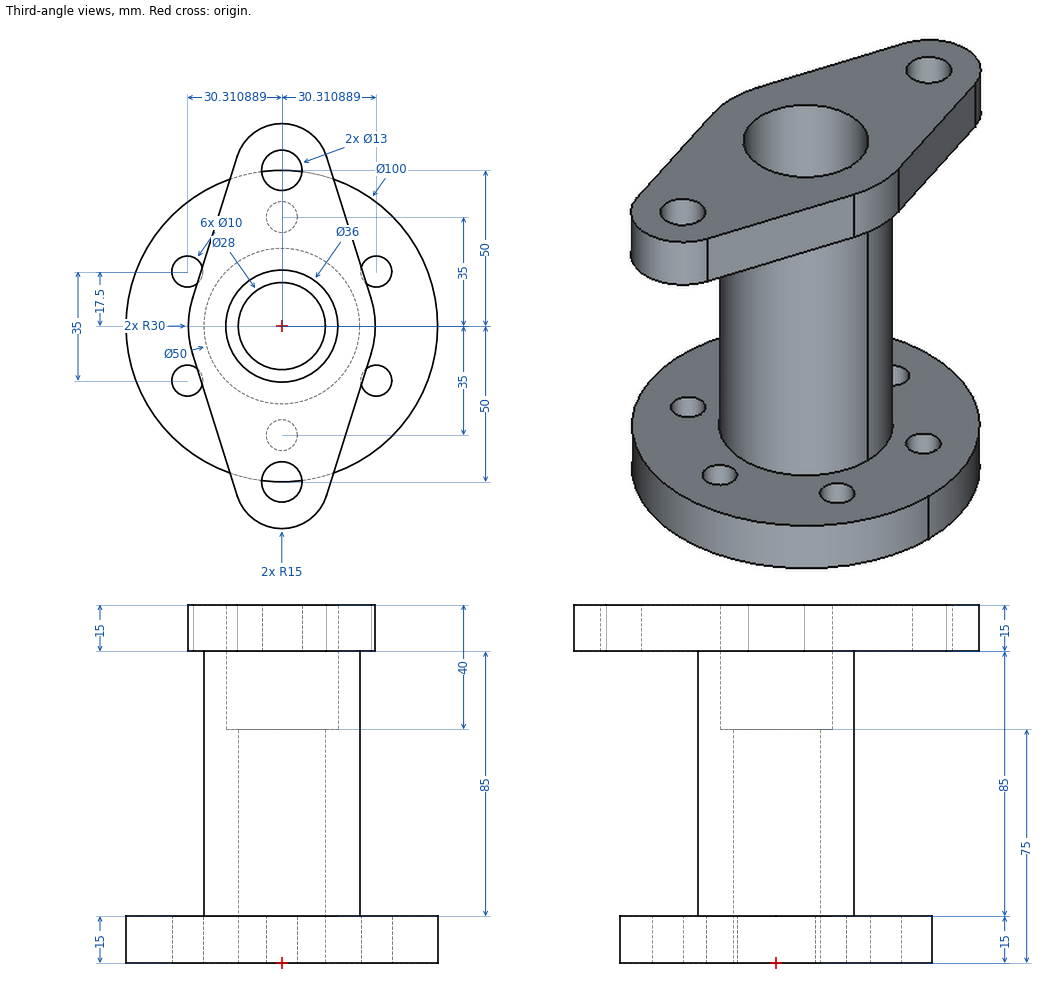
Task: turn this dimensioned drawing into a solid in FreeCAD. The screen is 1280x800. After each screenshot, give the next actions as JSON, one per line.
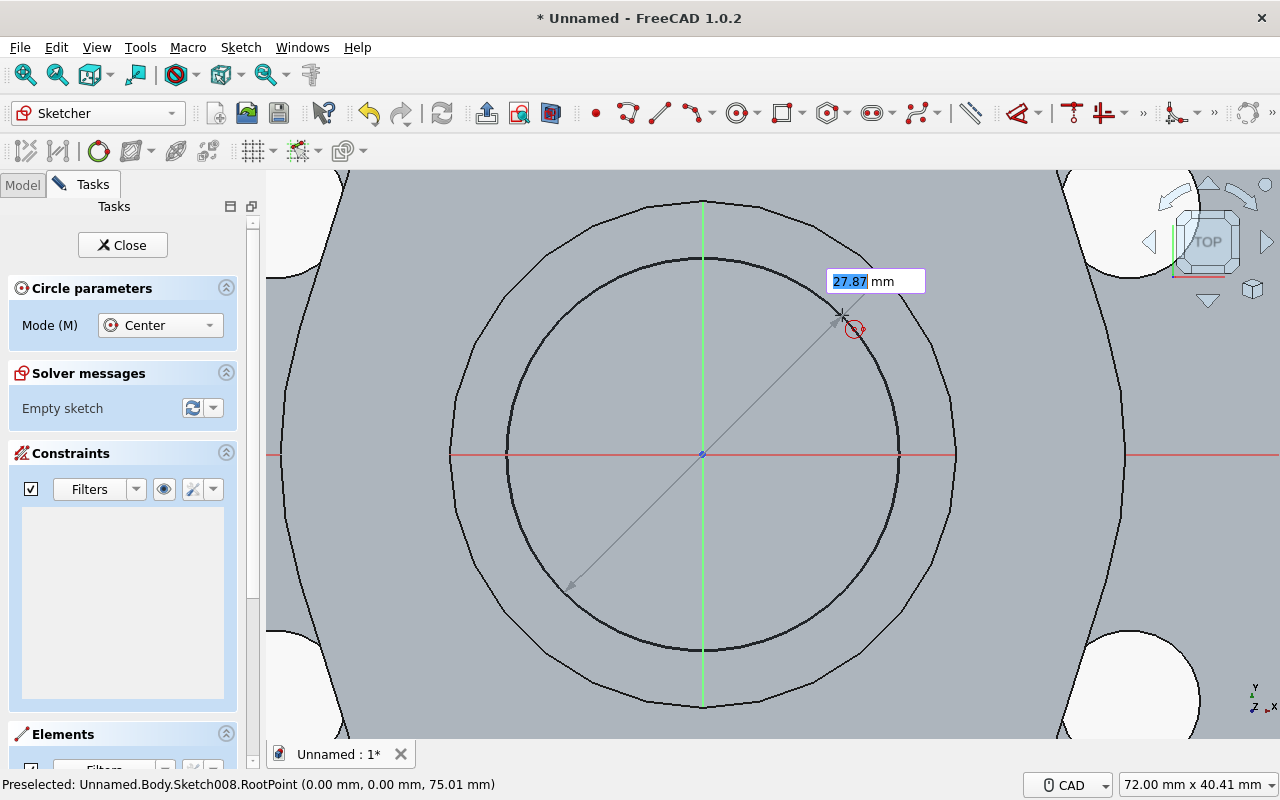
{"action": "type", "text": "28"}
{"action": "key", "text": "Return"}
{"action": "key", "text": "Escape"}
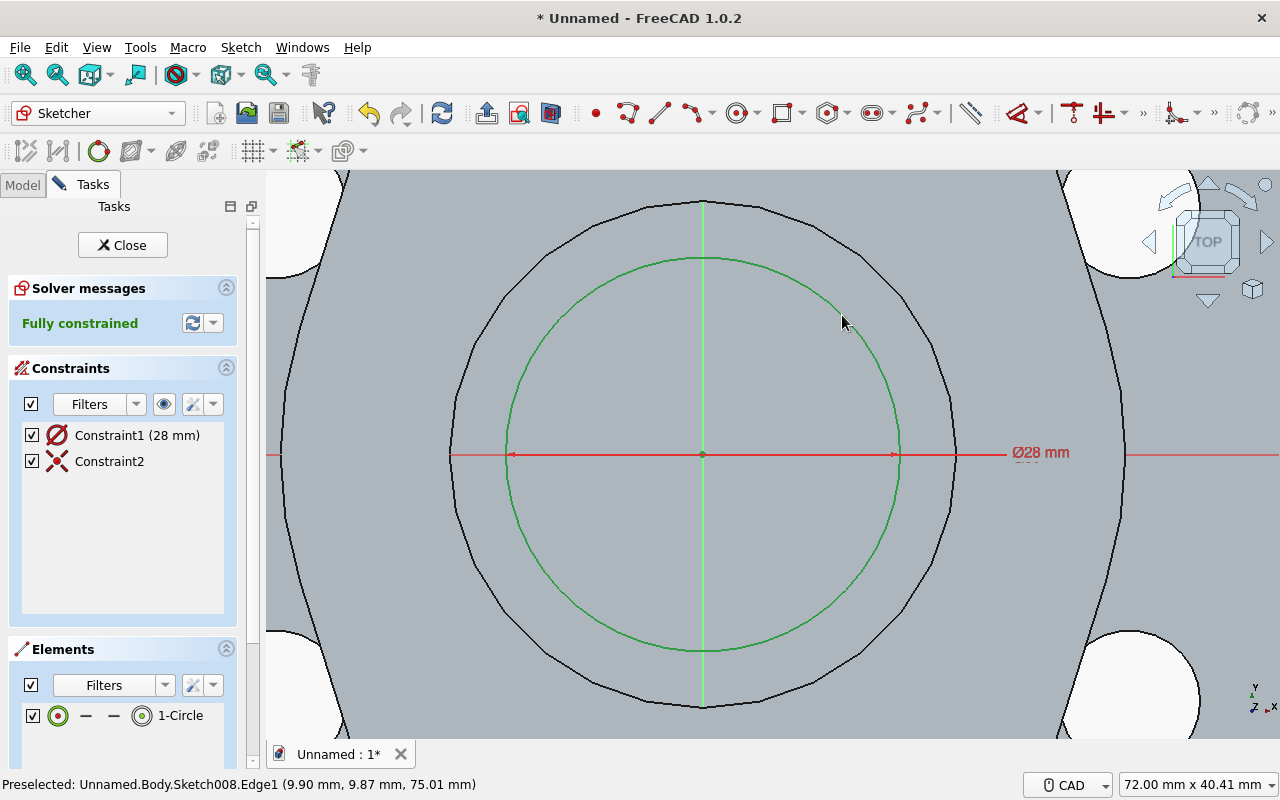
{"action": "left_click", "coordinate": [123, 245]}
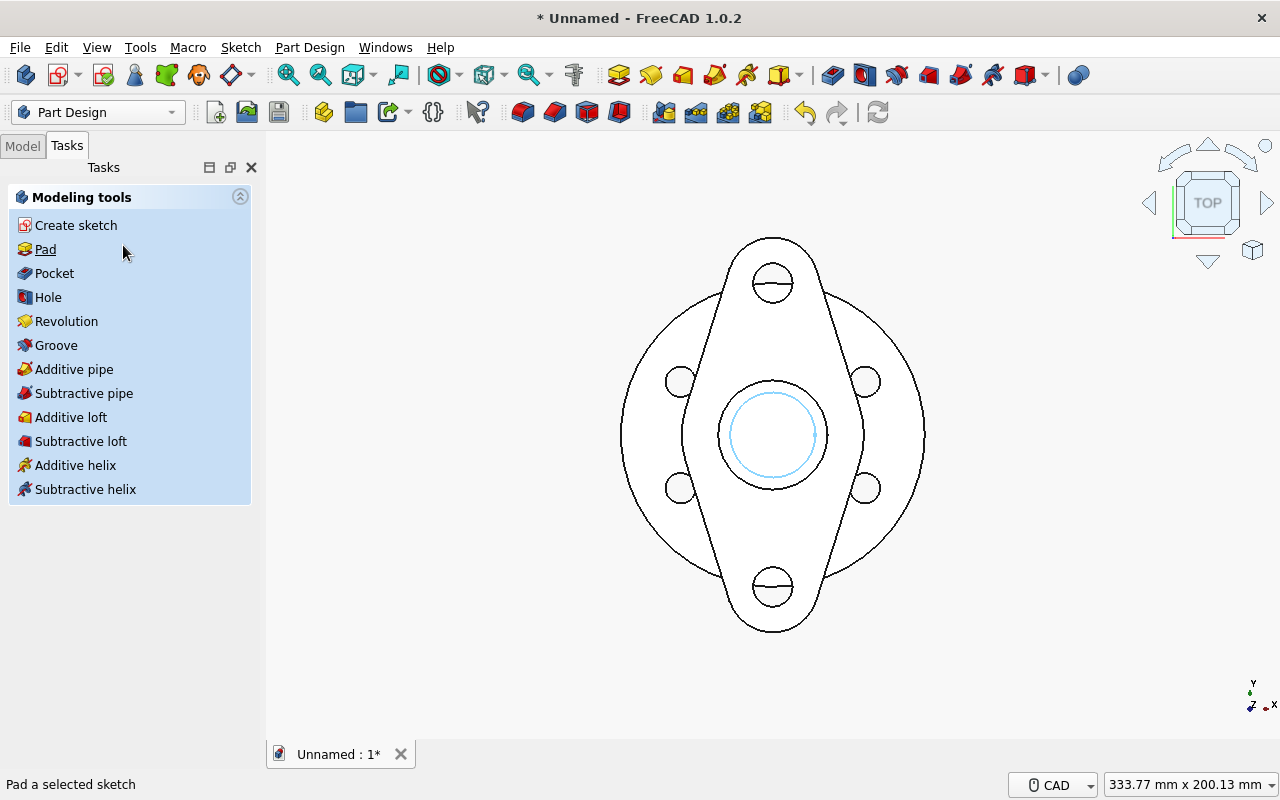
{"action": "left_click", "coordinate": [834, 76]}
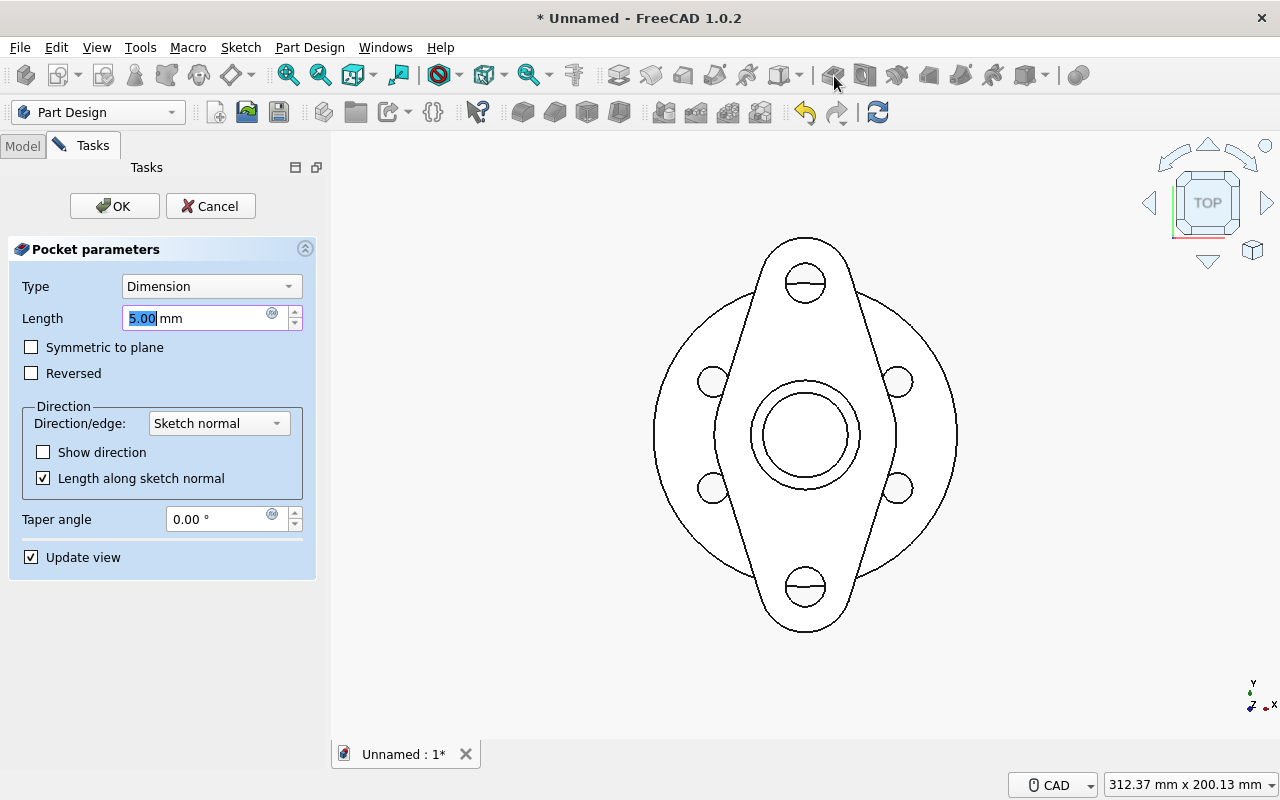
{"action": "type", "text": "75"}
{"action": "key", "text": "Tab"}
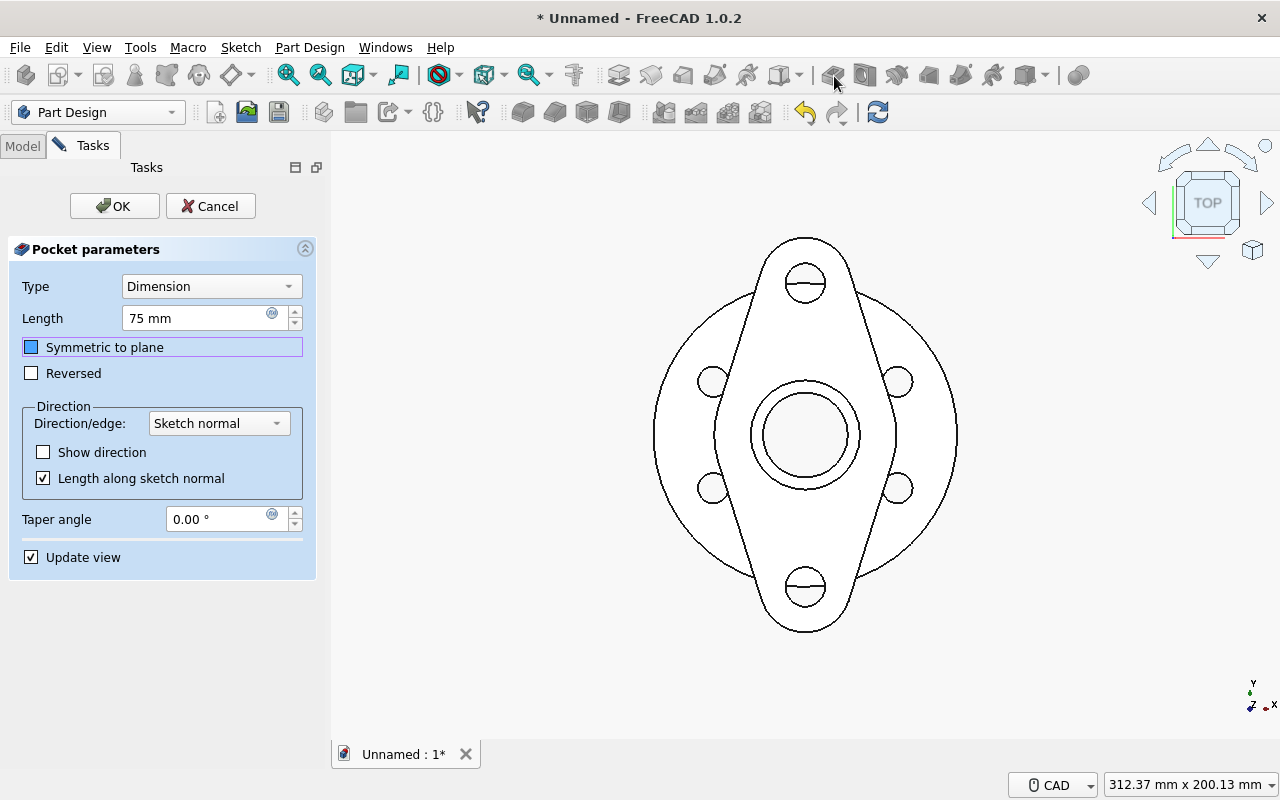
{"action": "left_click", "coordinate": [115, 206]}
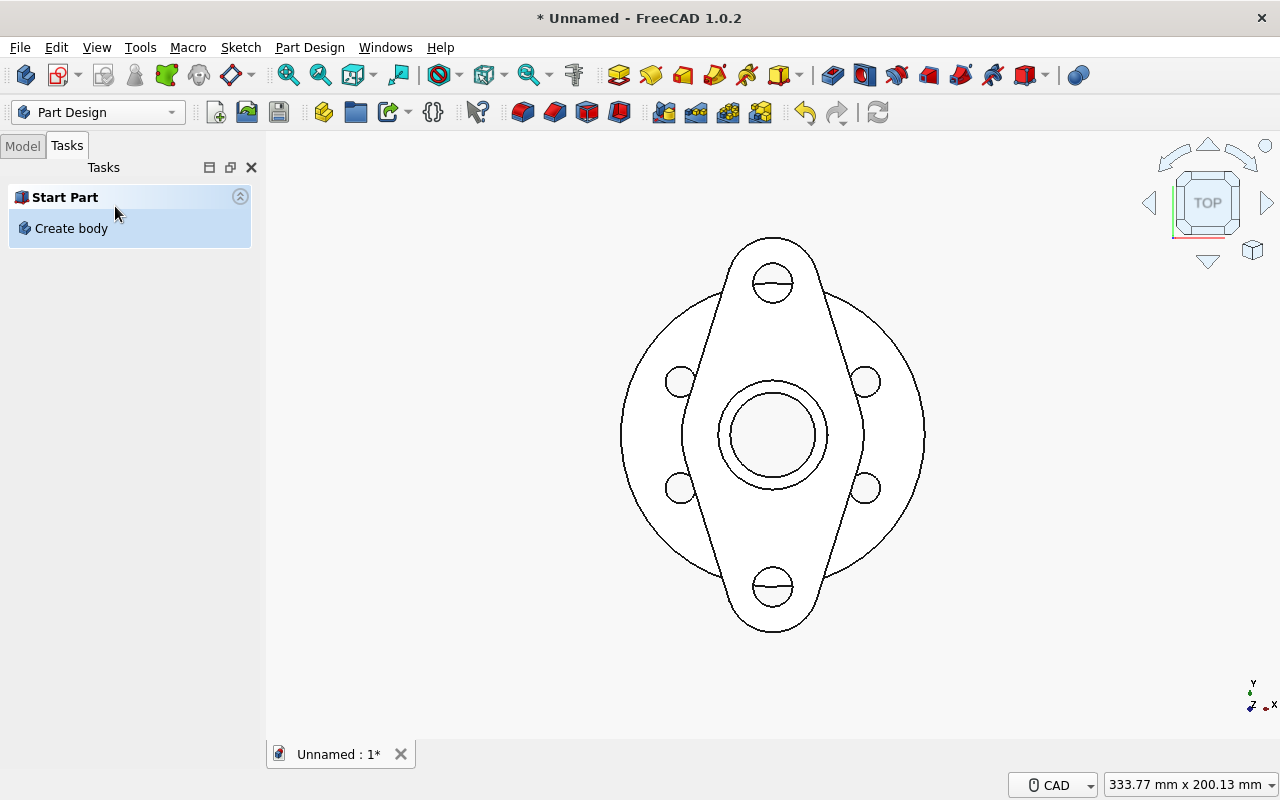
{"action": "key", "text": "0"}